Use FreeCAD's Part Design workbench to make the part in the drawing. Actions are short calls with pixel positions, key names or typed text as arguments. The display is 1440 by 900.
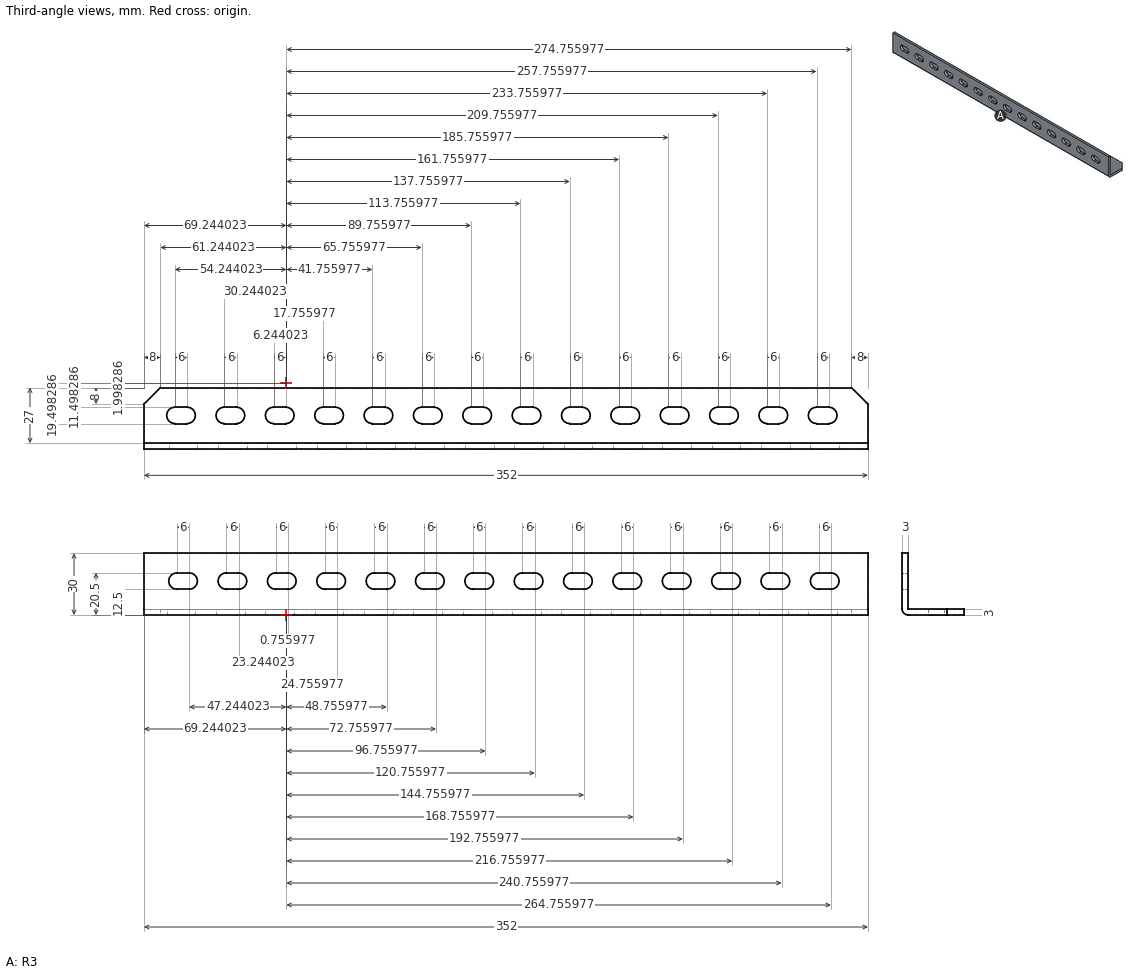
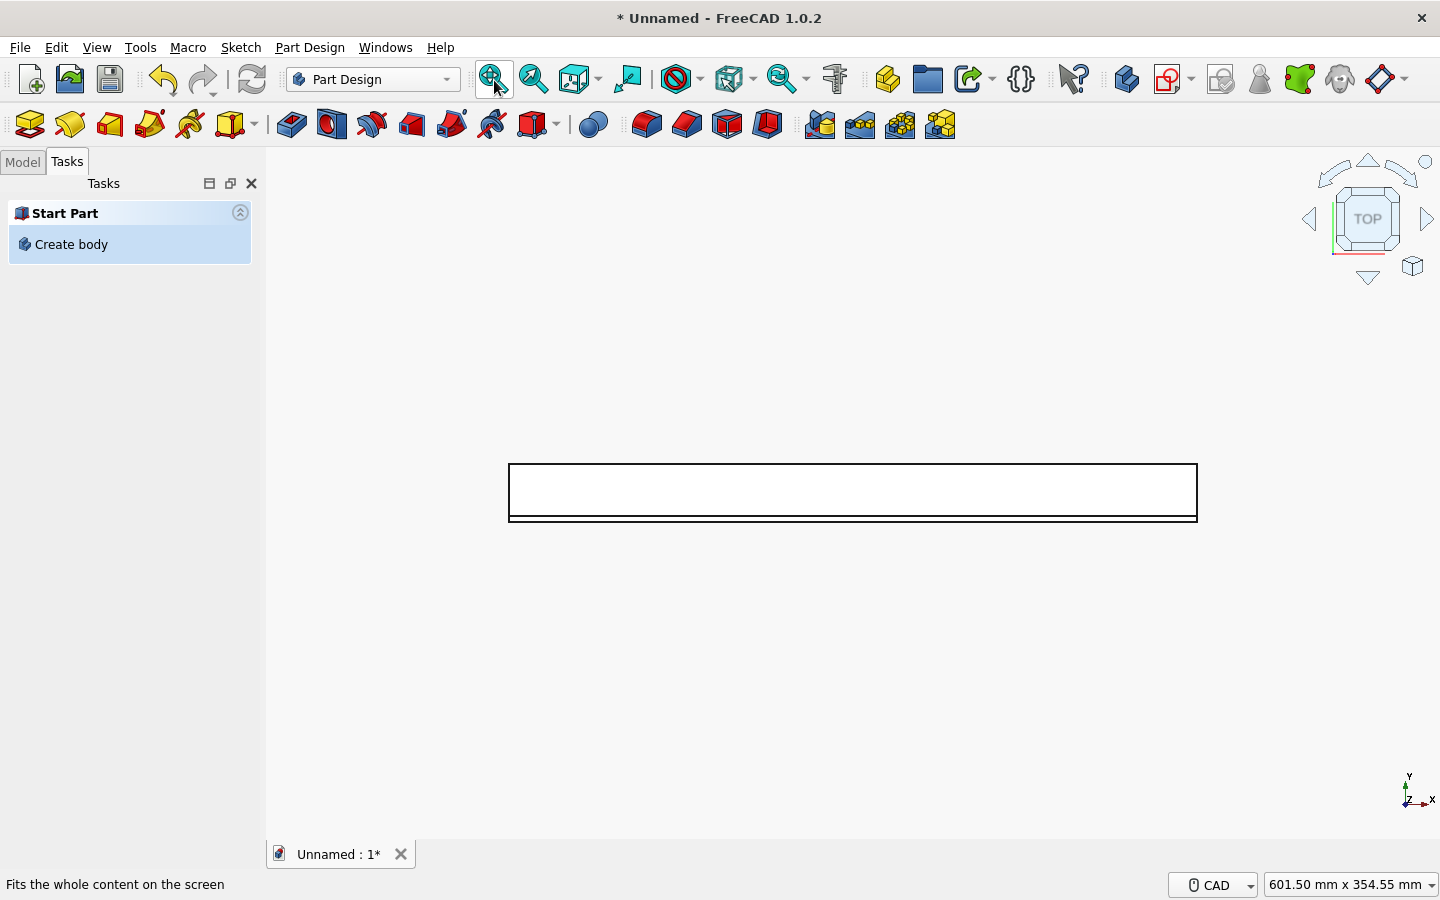
key(1)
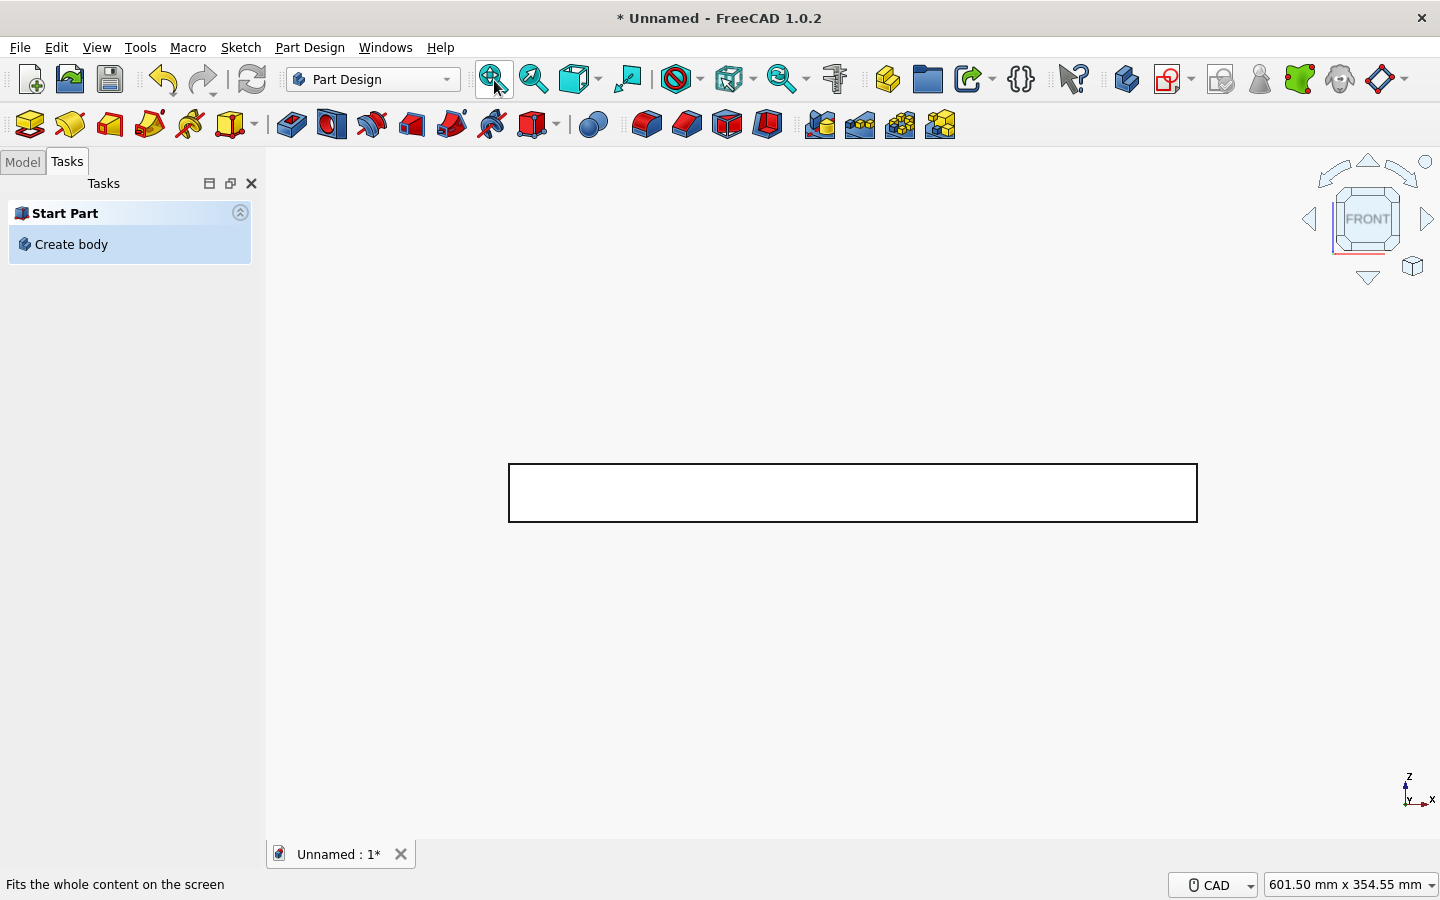
click(853, 521)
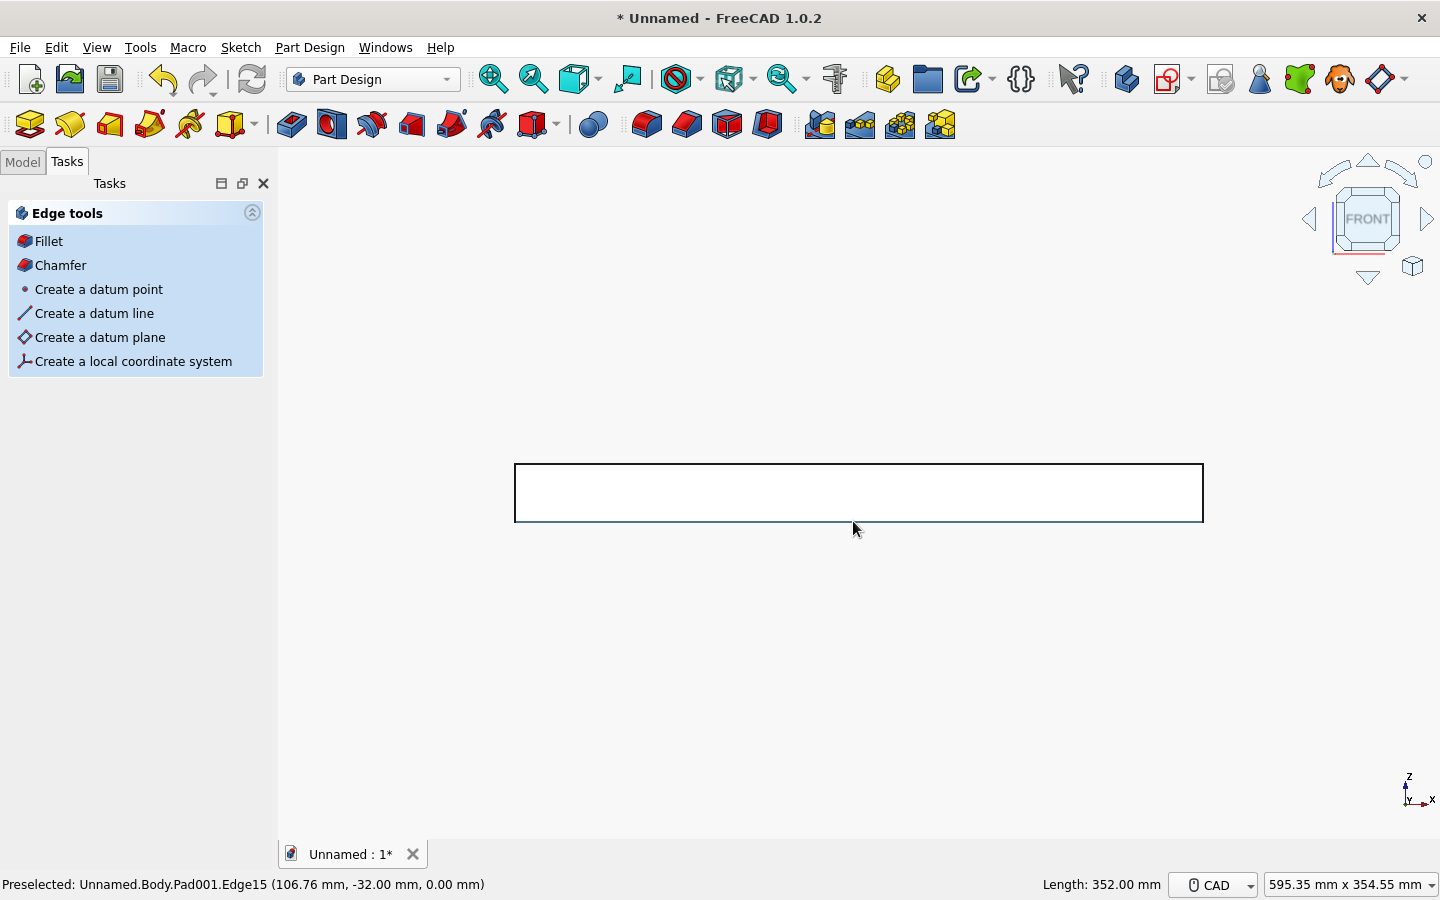
click(648, 124)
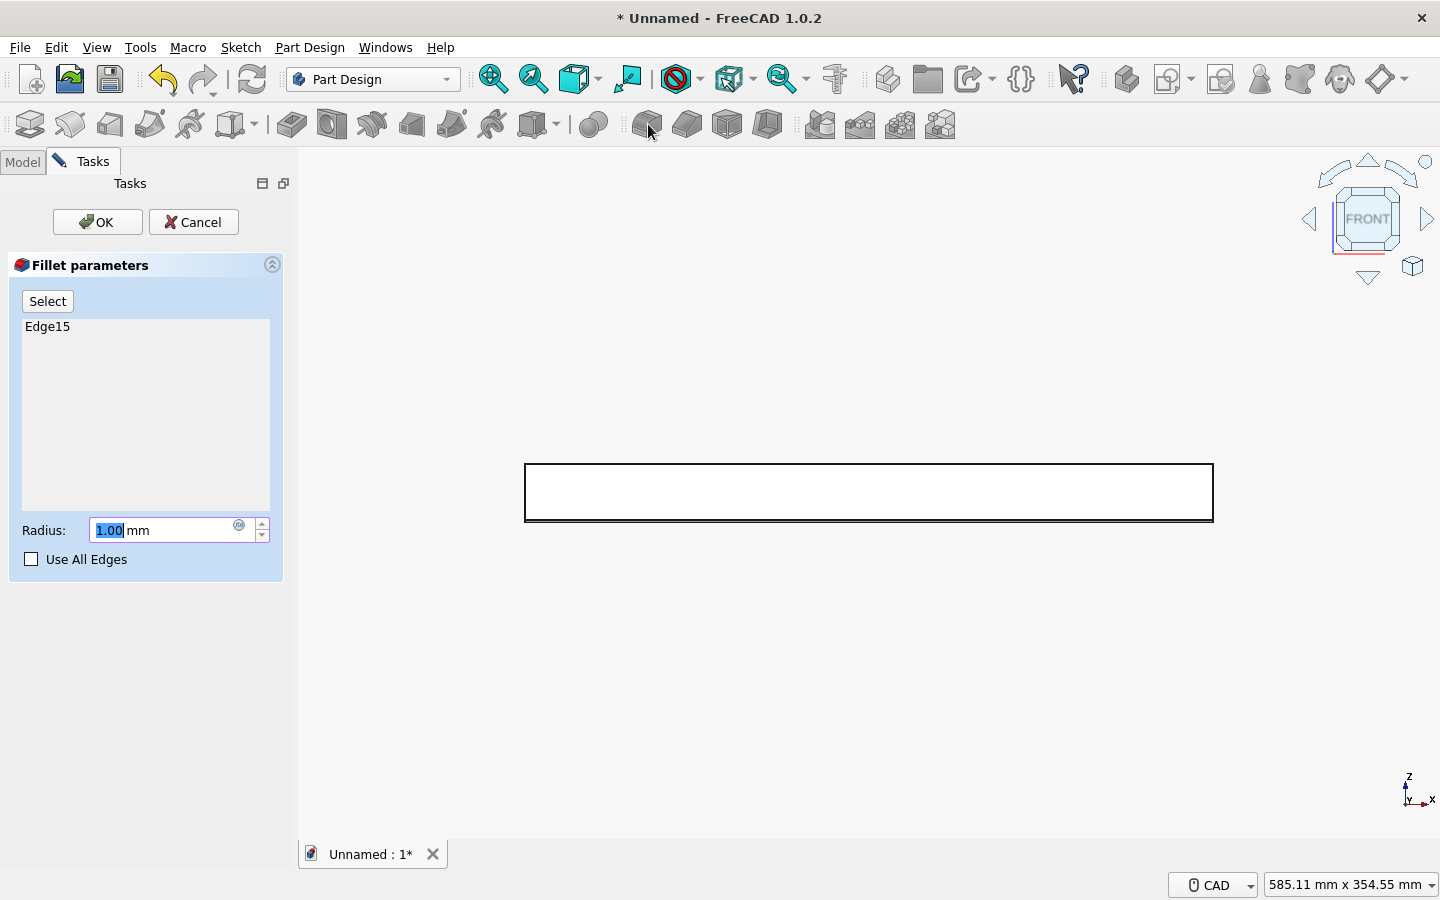
text(3)
key(Tab)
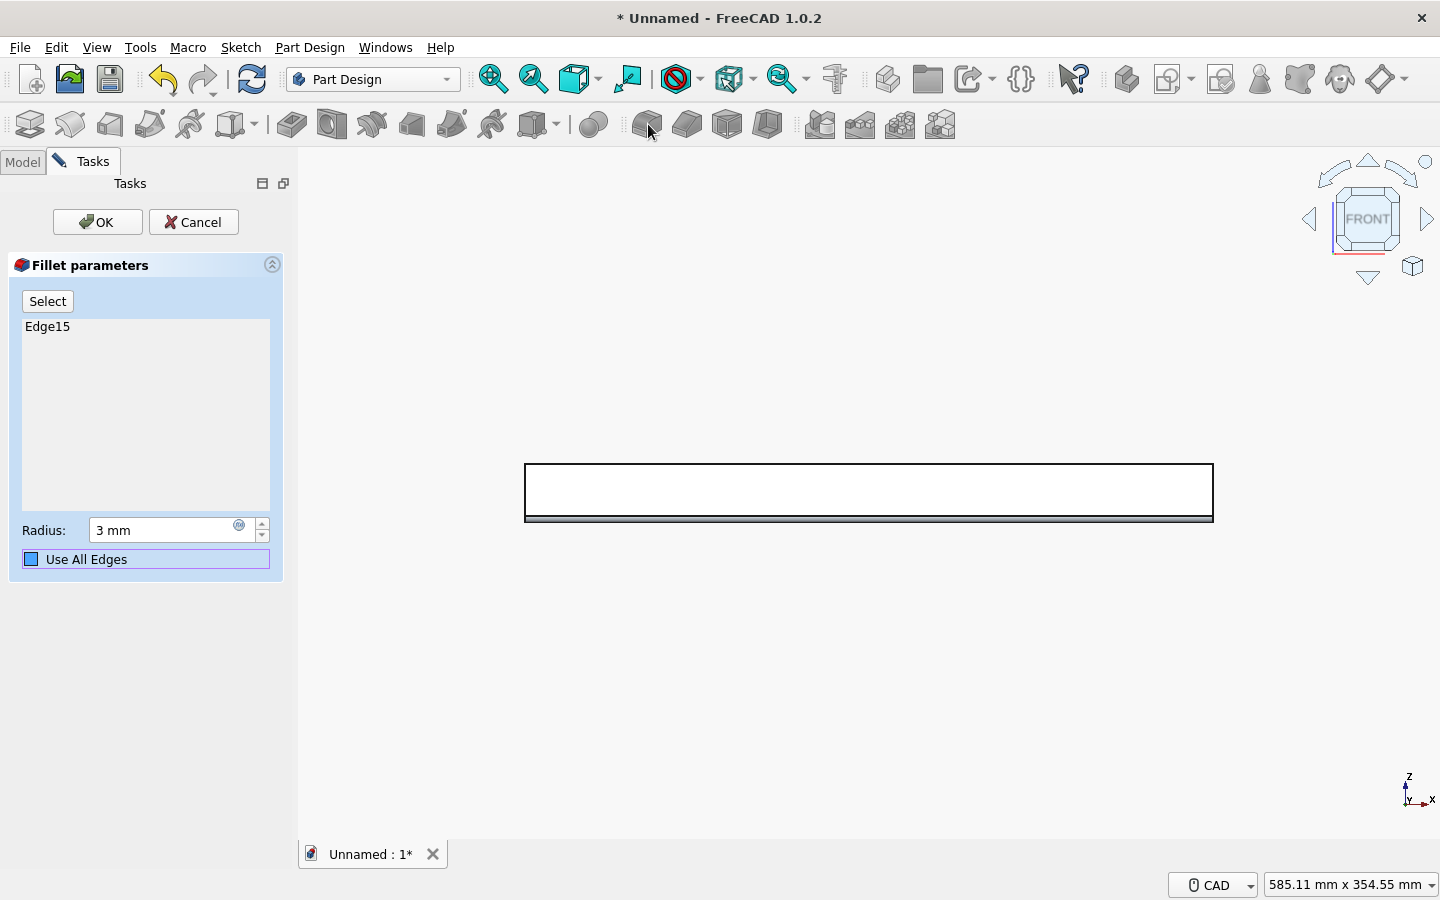
click(98, 222)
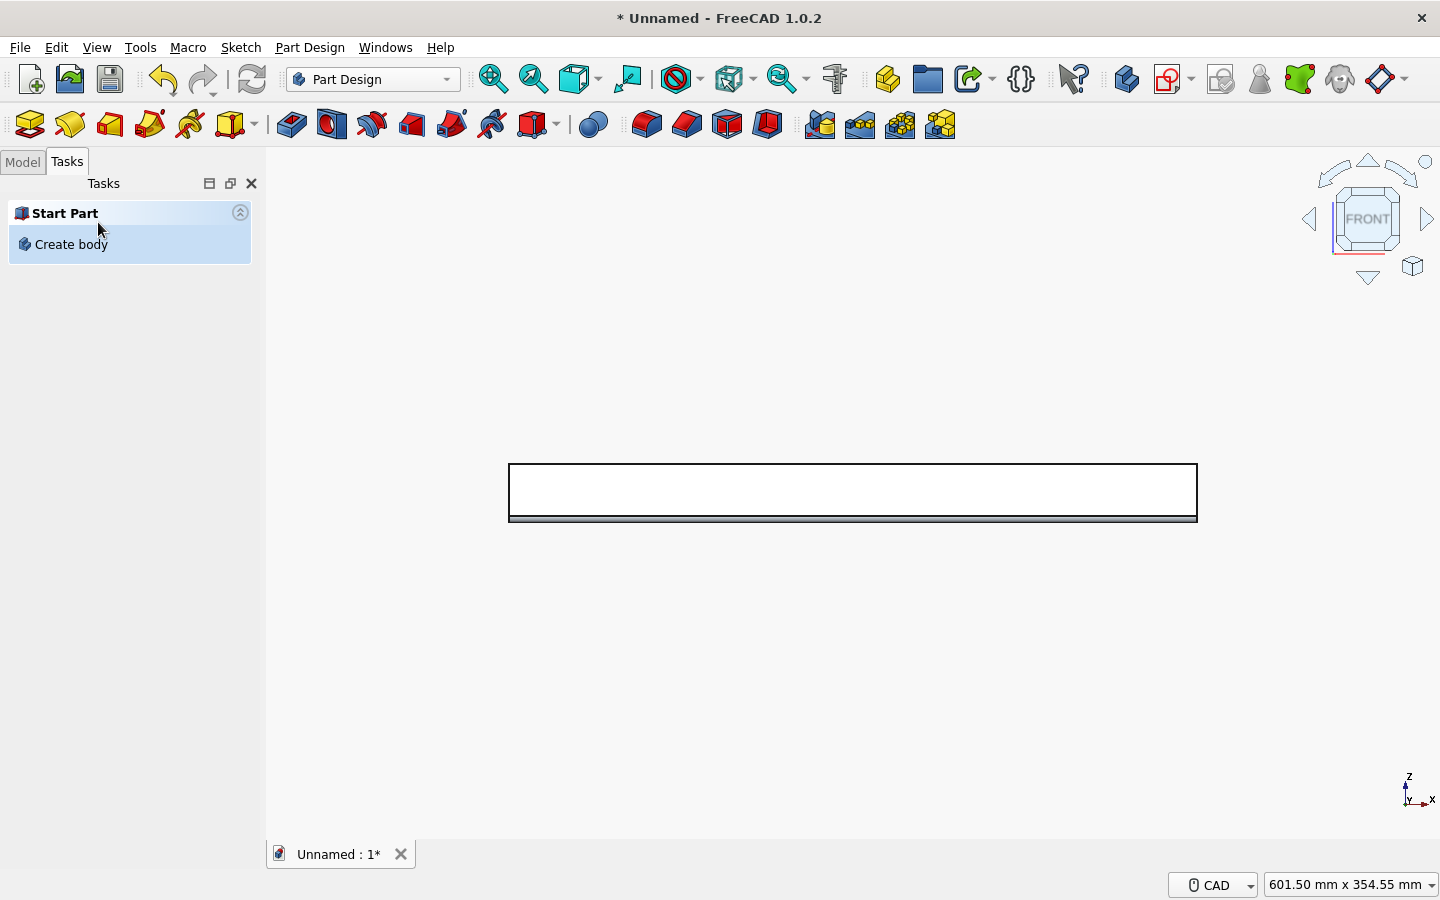
key(4)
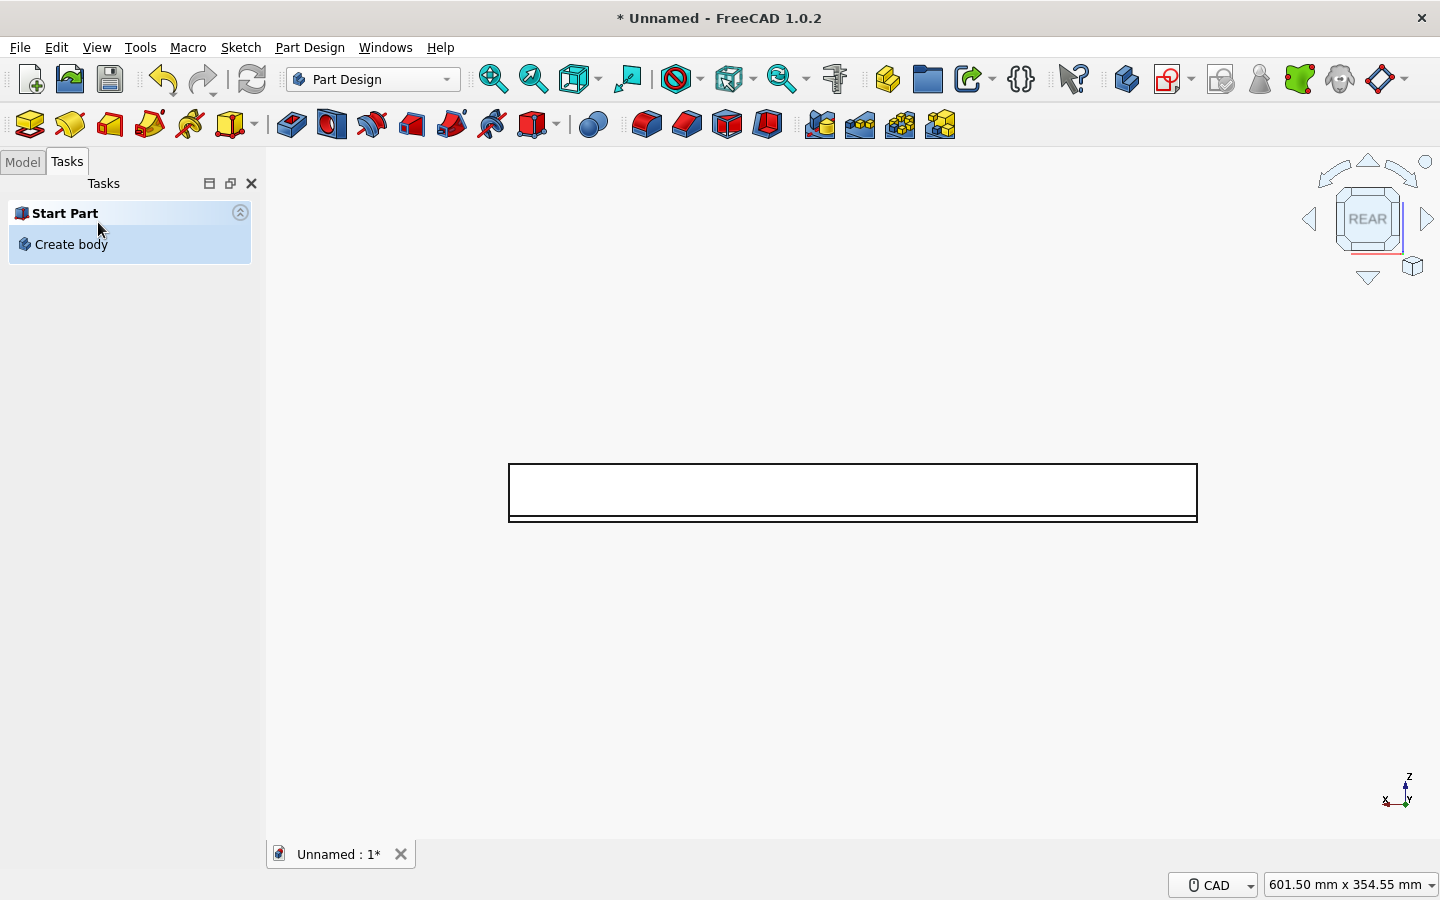
click(559, 489)